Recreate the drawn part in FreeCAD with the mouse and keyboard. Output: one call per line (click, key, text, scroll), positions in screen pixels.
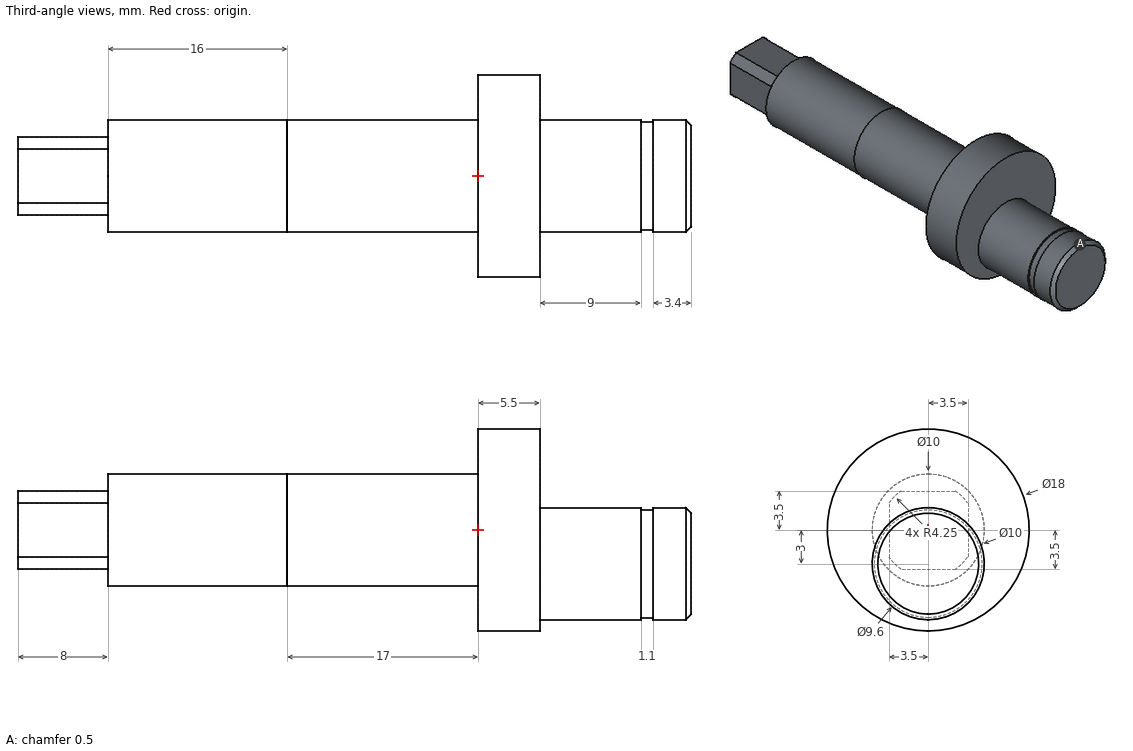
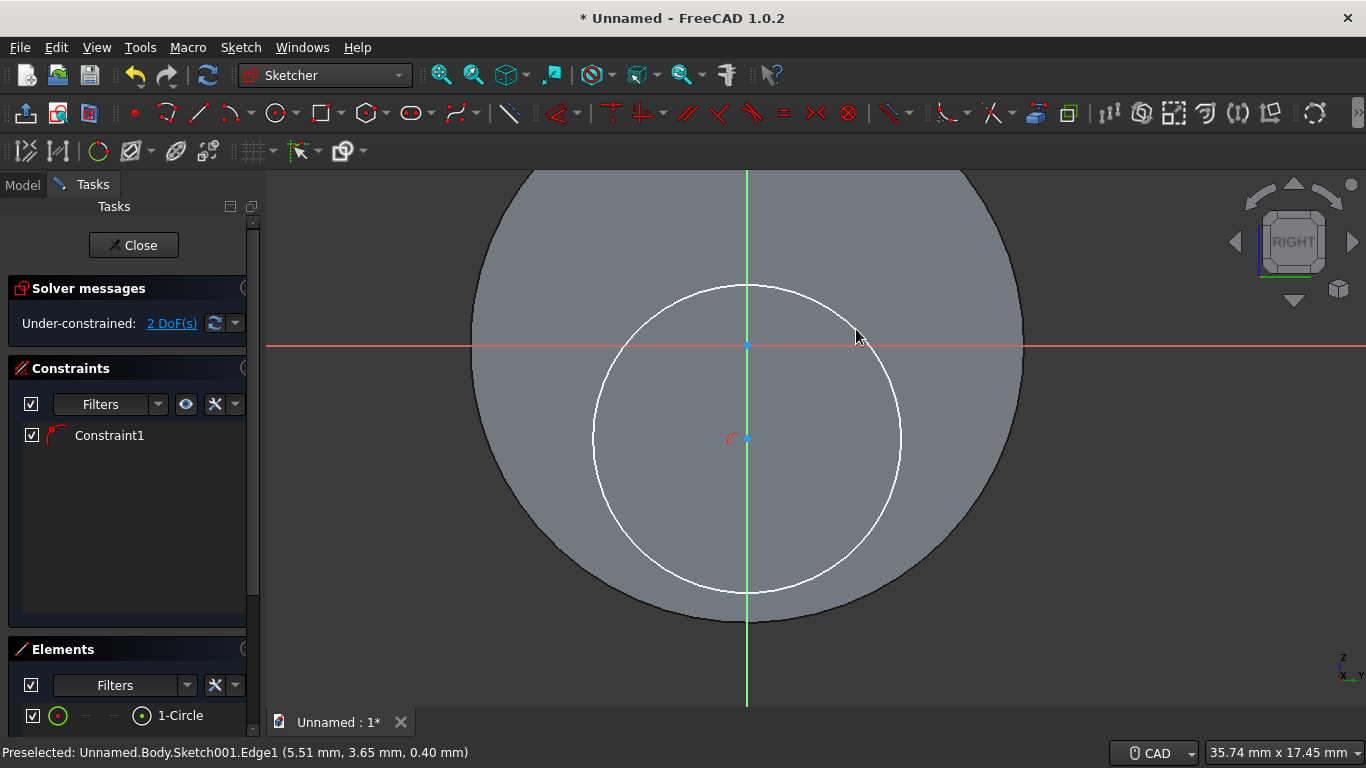
click(556, 114)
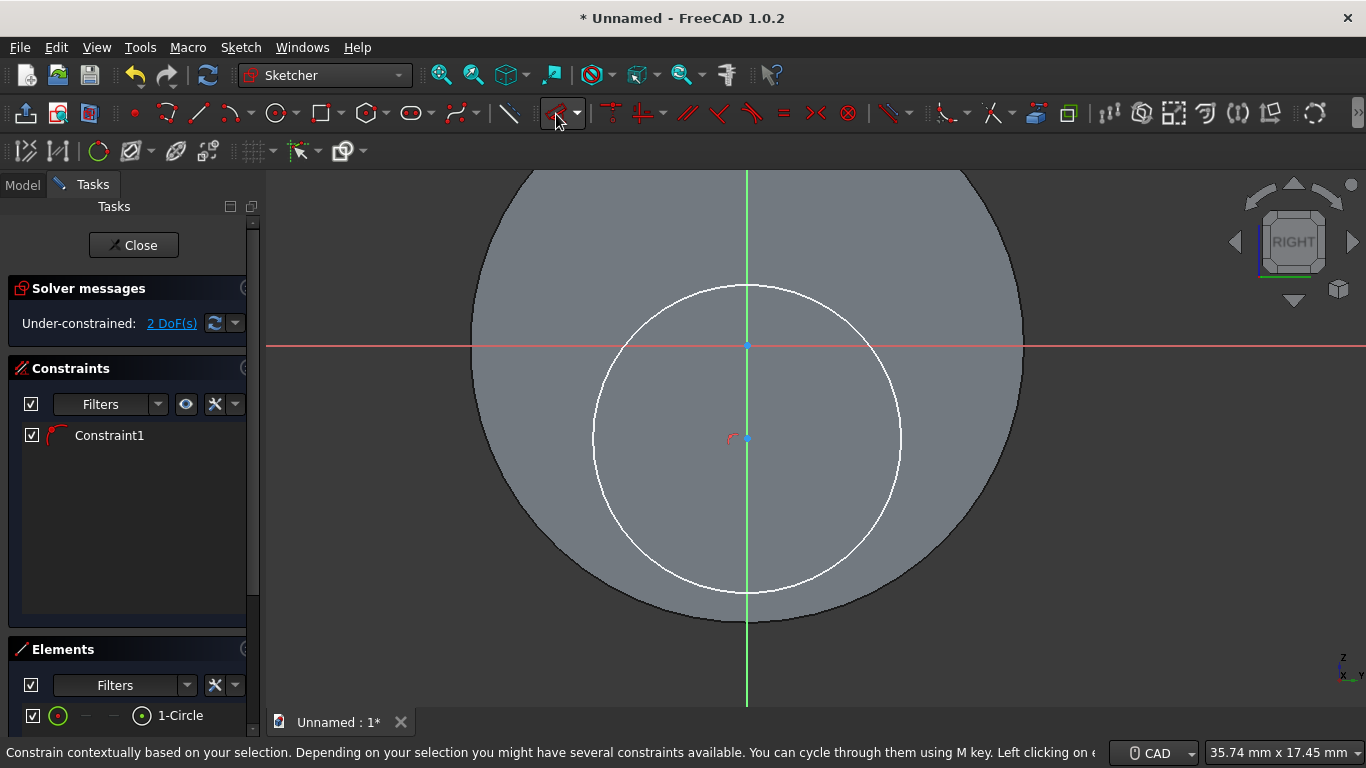
click(856, 330)
click(879, 307)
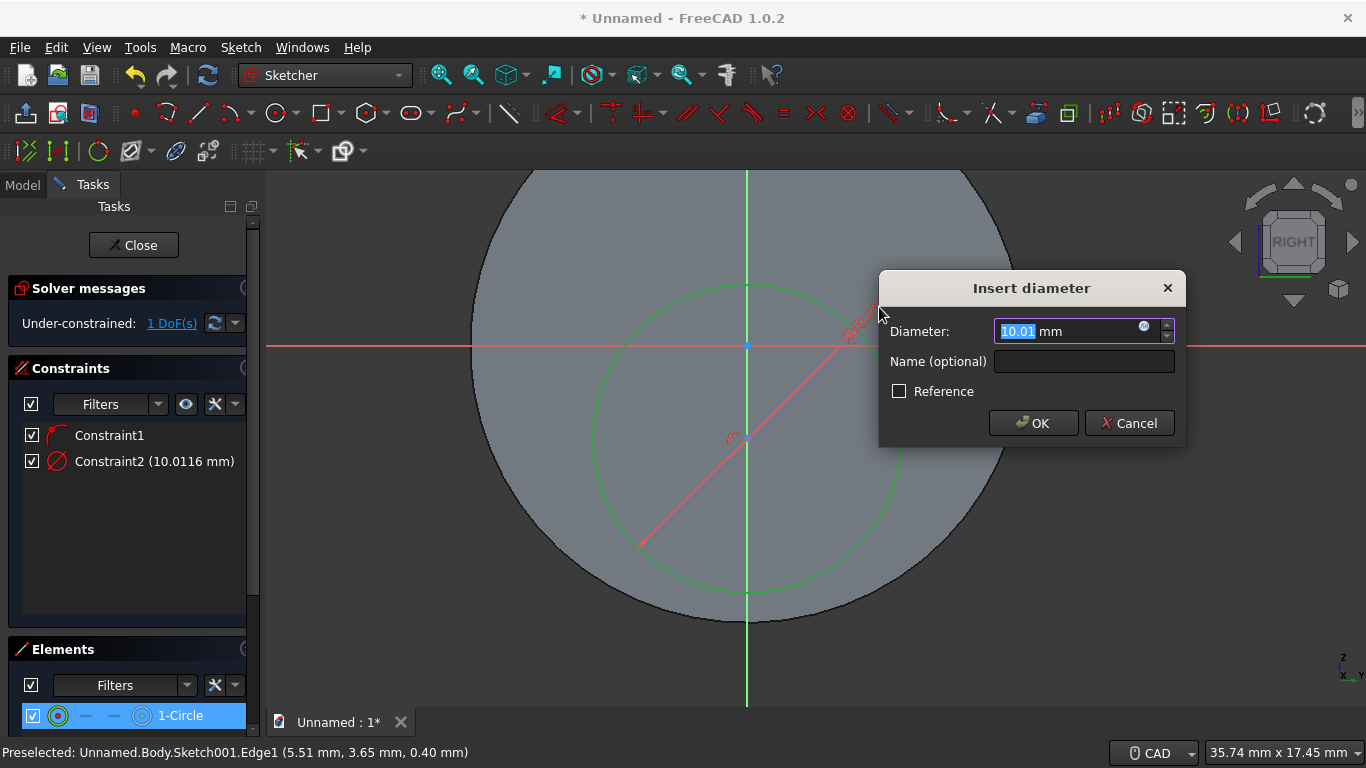
text(10)
key(Return)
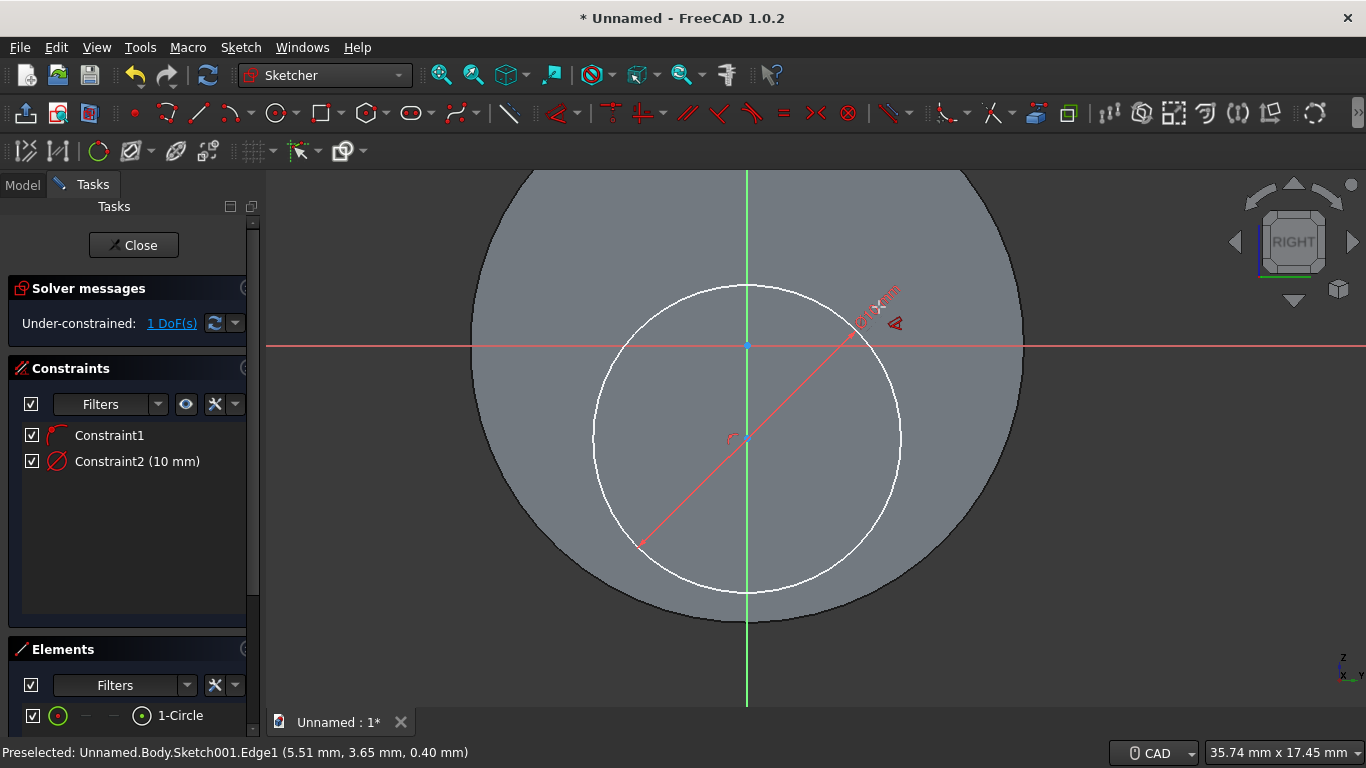
click(747, 439)
click(781, 392)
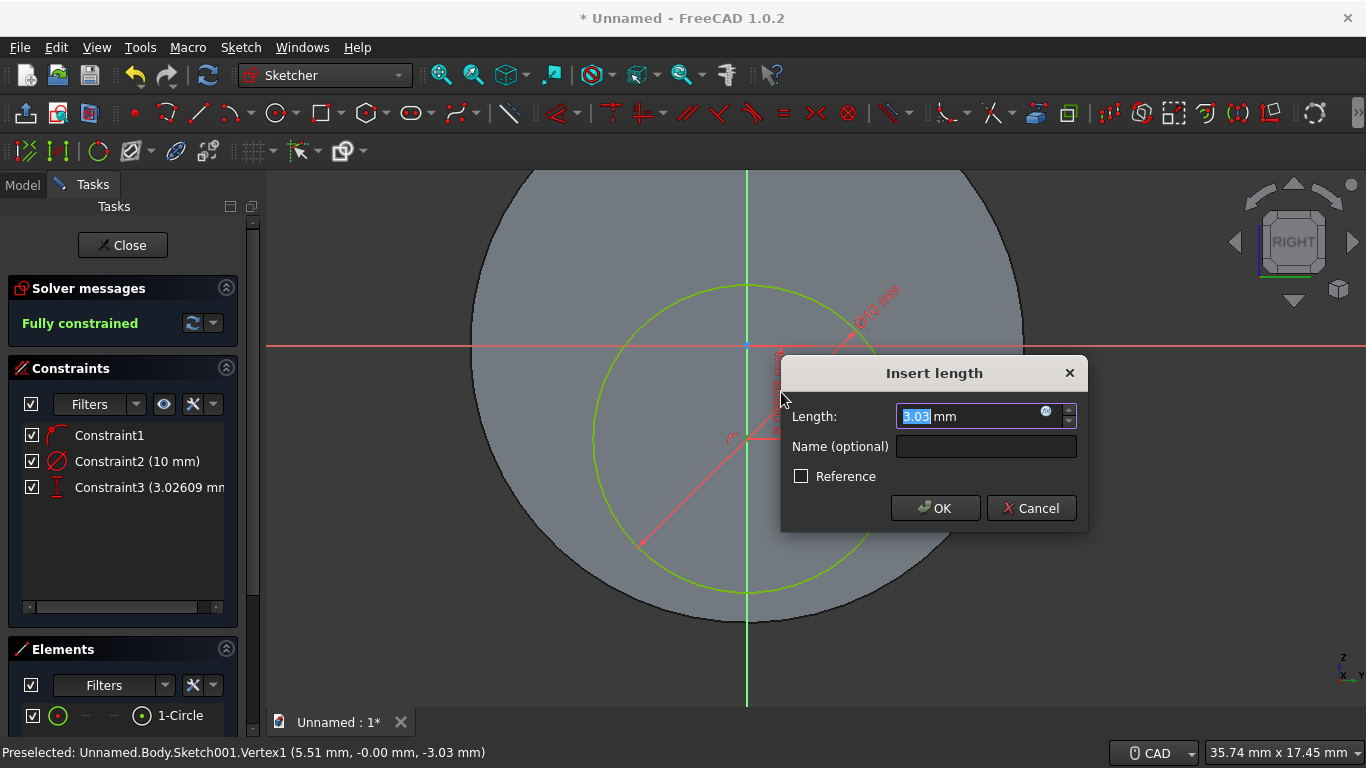
text(3)
key(Return)
key(Escape)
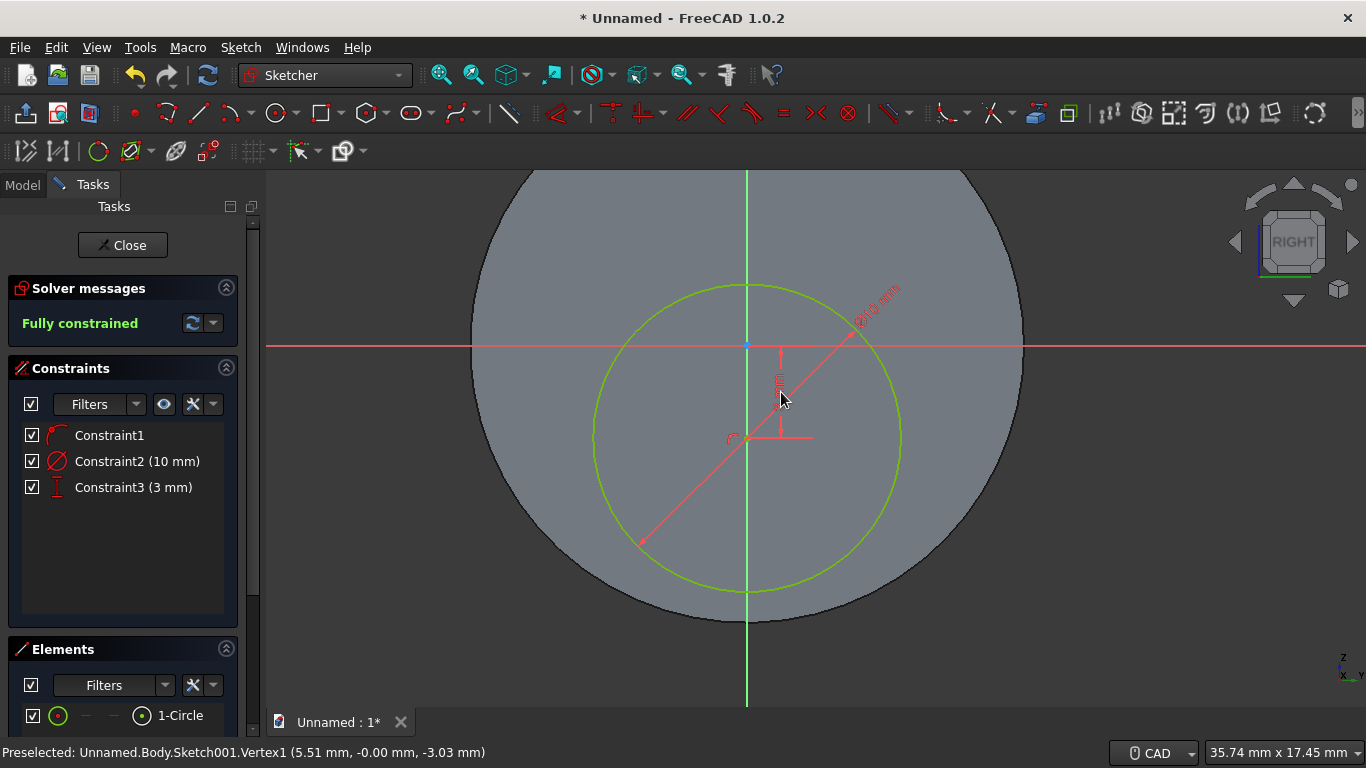
click(123, 245)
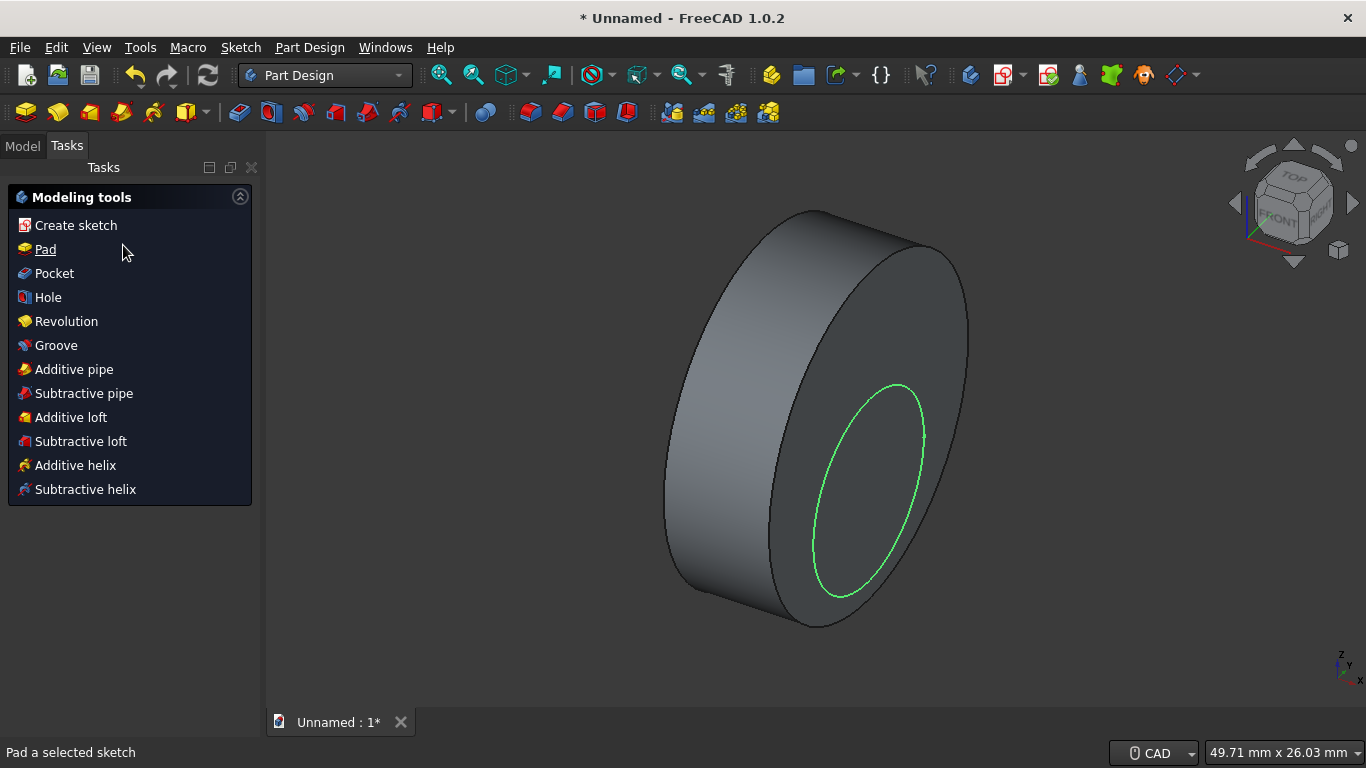
click(26, 112)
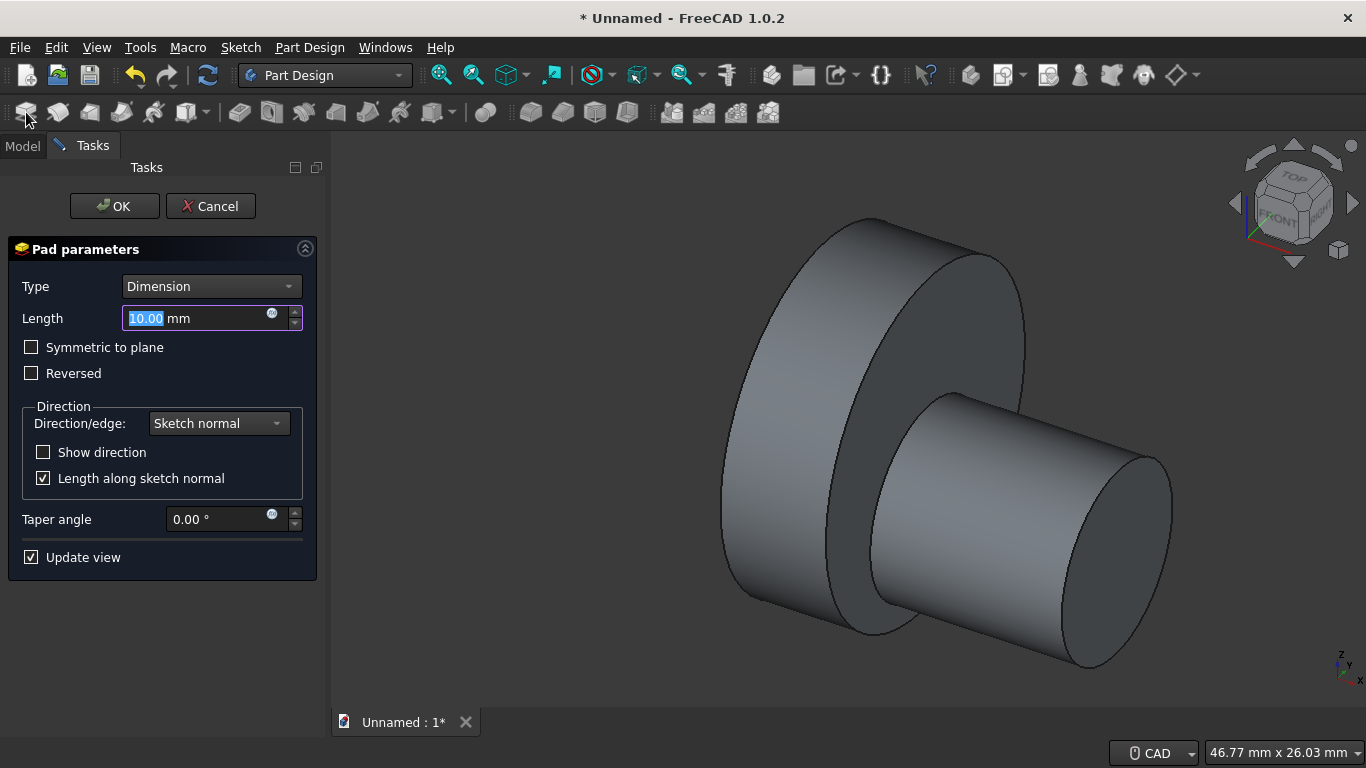
text(9)
key(Tab)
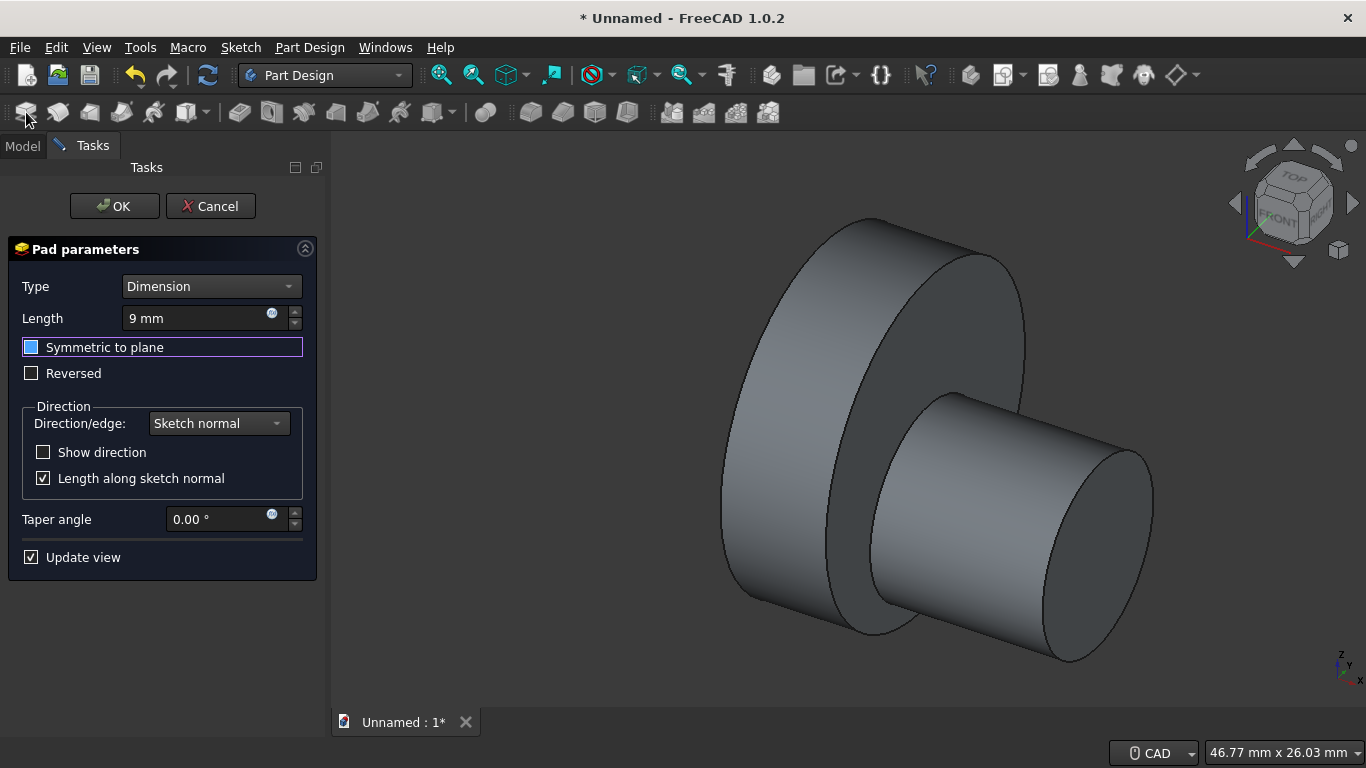
click(115, 206)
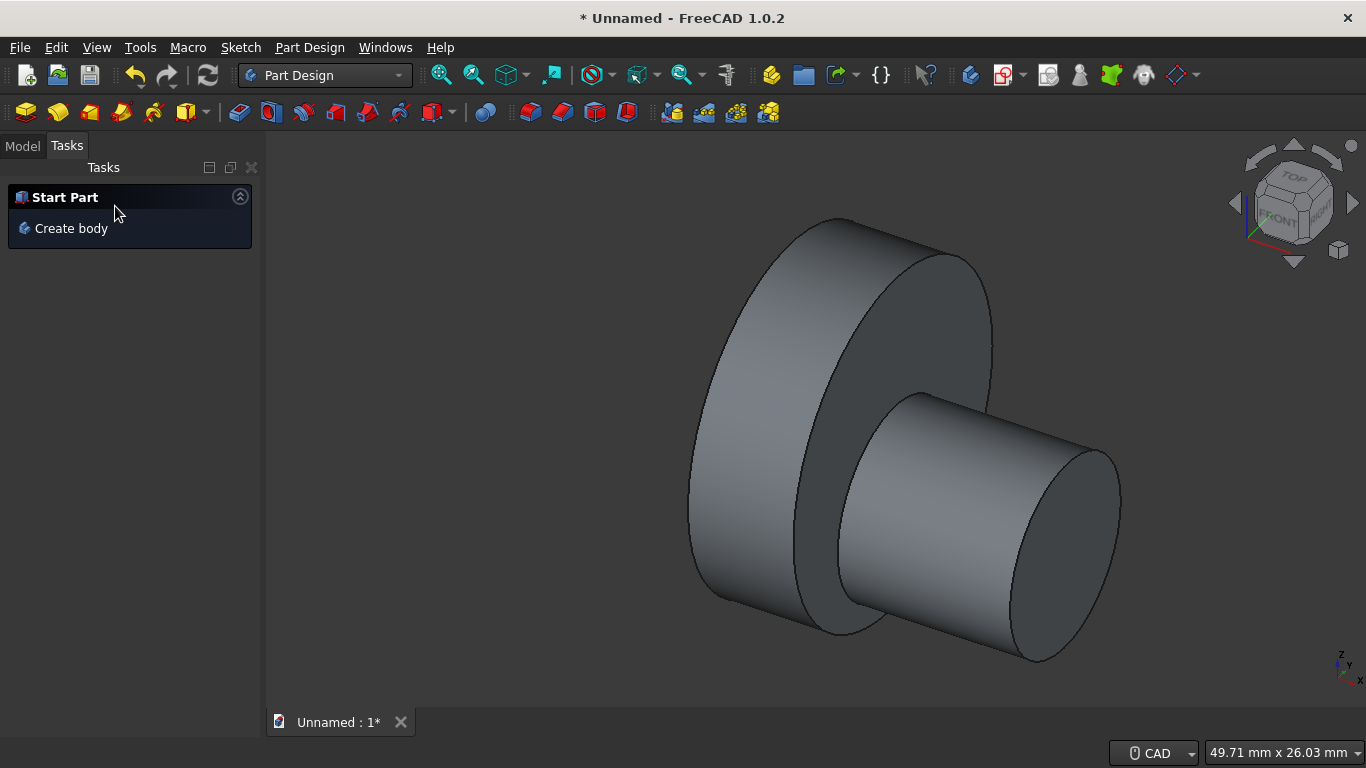
click(442, 76)